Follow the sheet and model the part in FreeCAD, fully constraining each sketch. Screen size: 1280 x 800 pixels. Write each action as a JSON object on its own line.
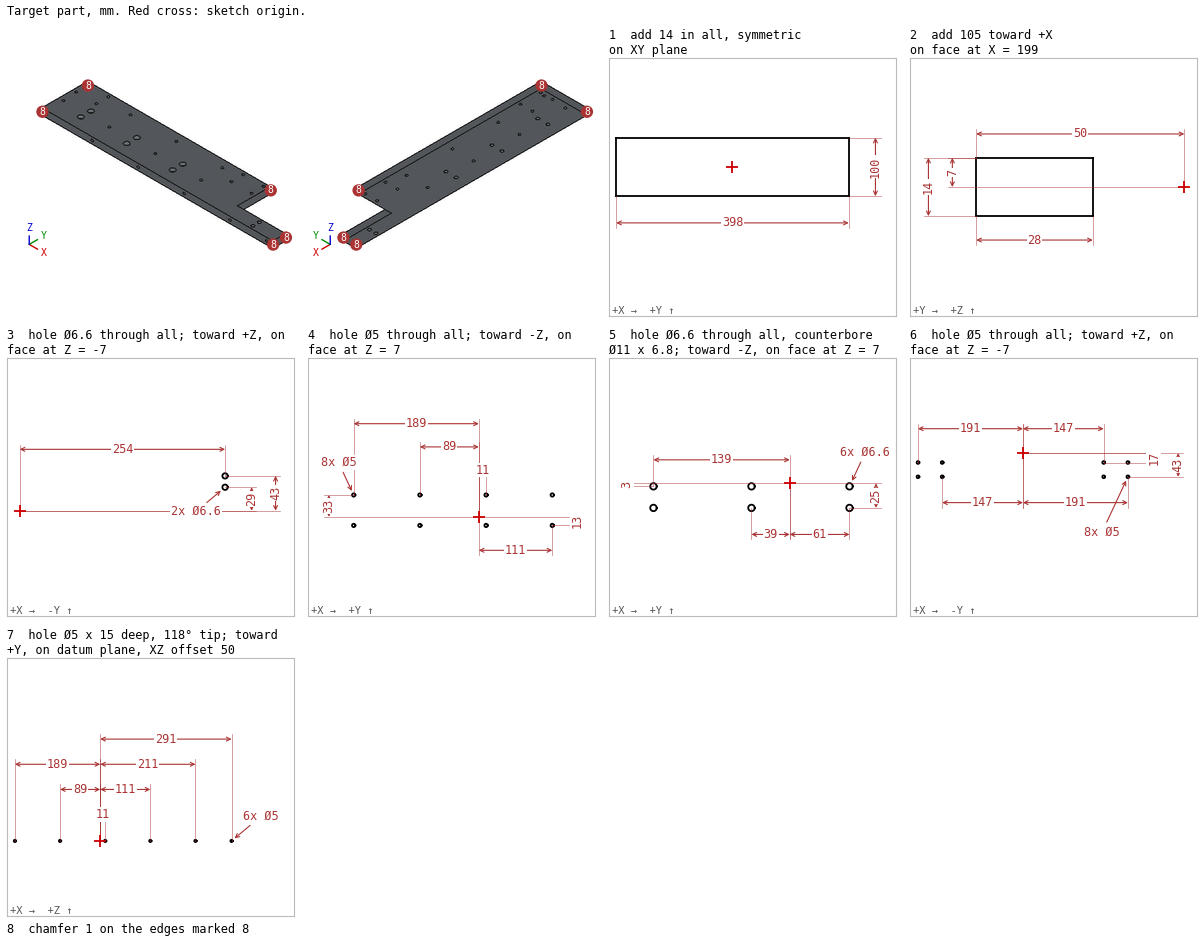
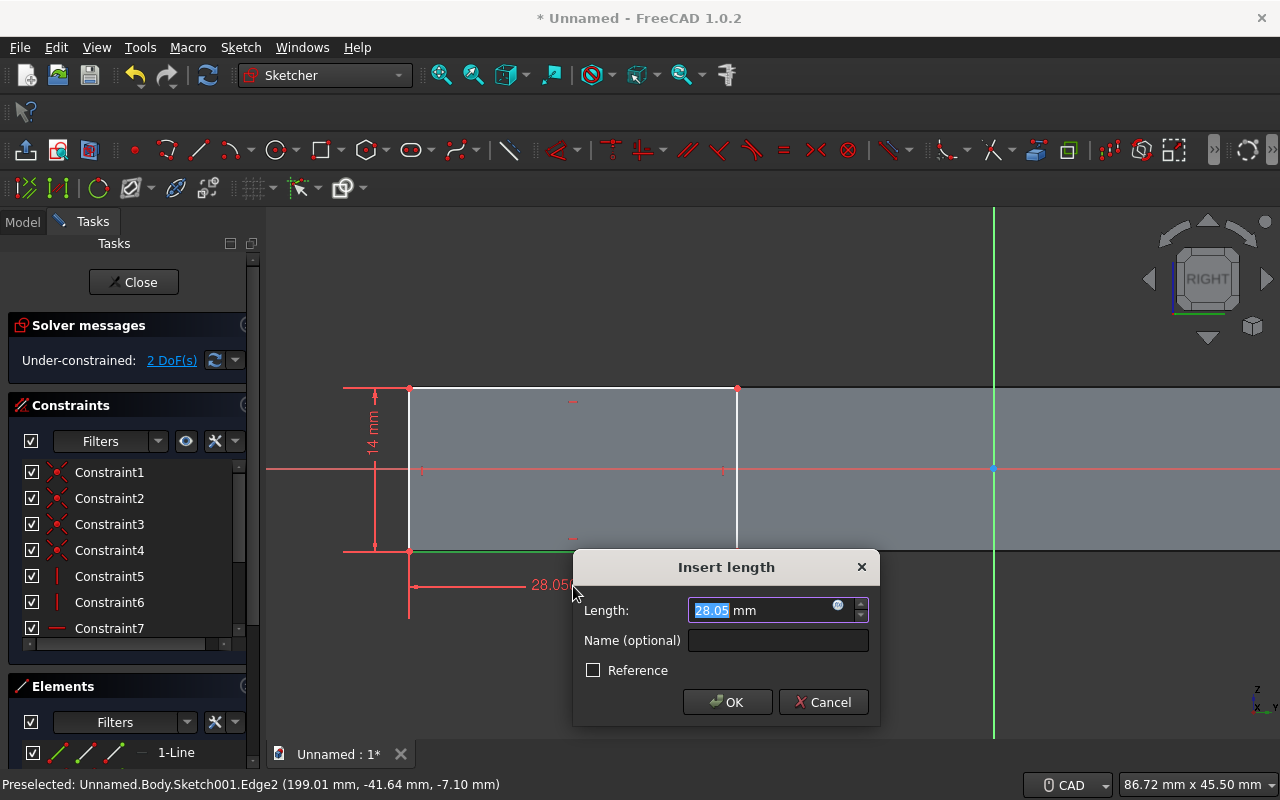
{"action": "type", "text": "28"}
{"action": "key", "text": "Return"}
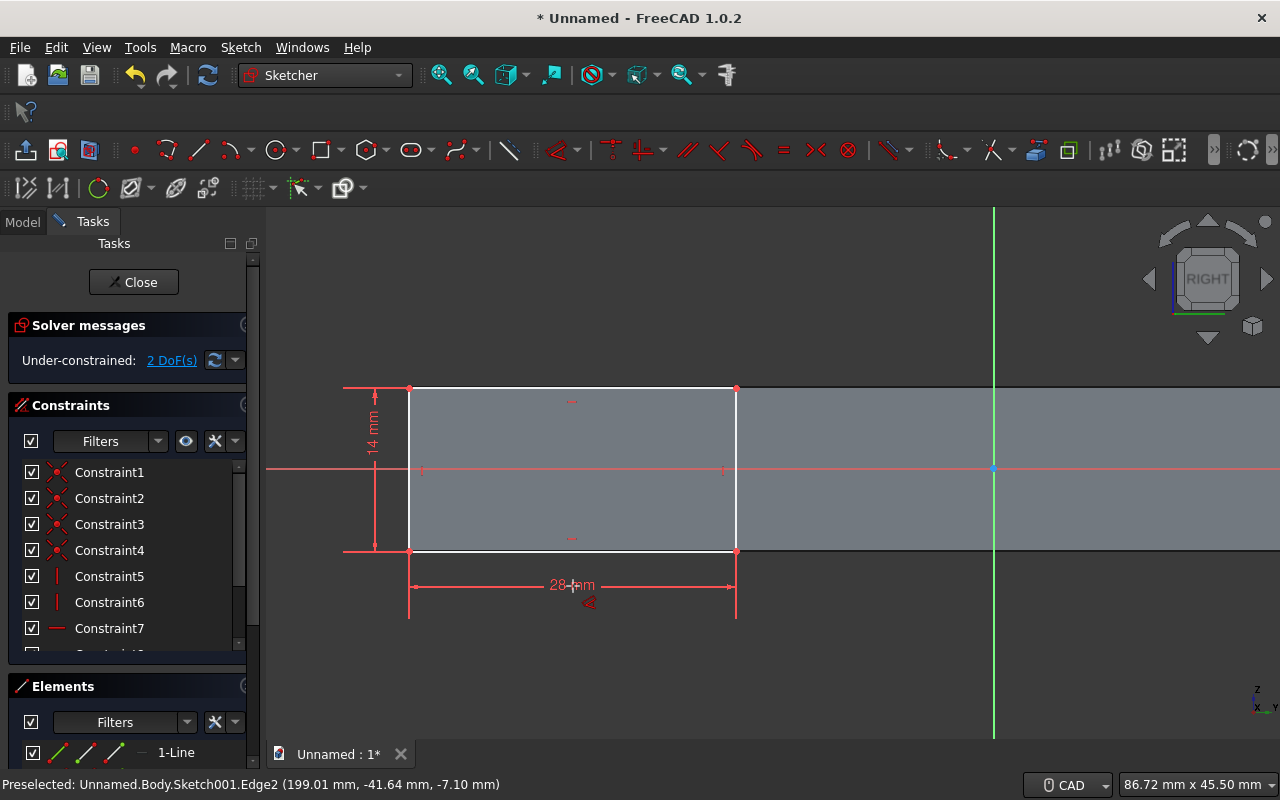
{"action": "left_click", "coordinate": [409, 388]}
{"action": "left_click", "coordinate": [375, 410]}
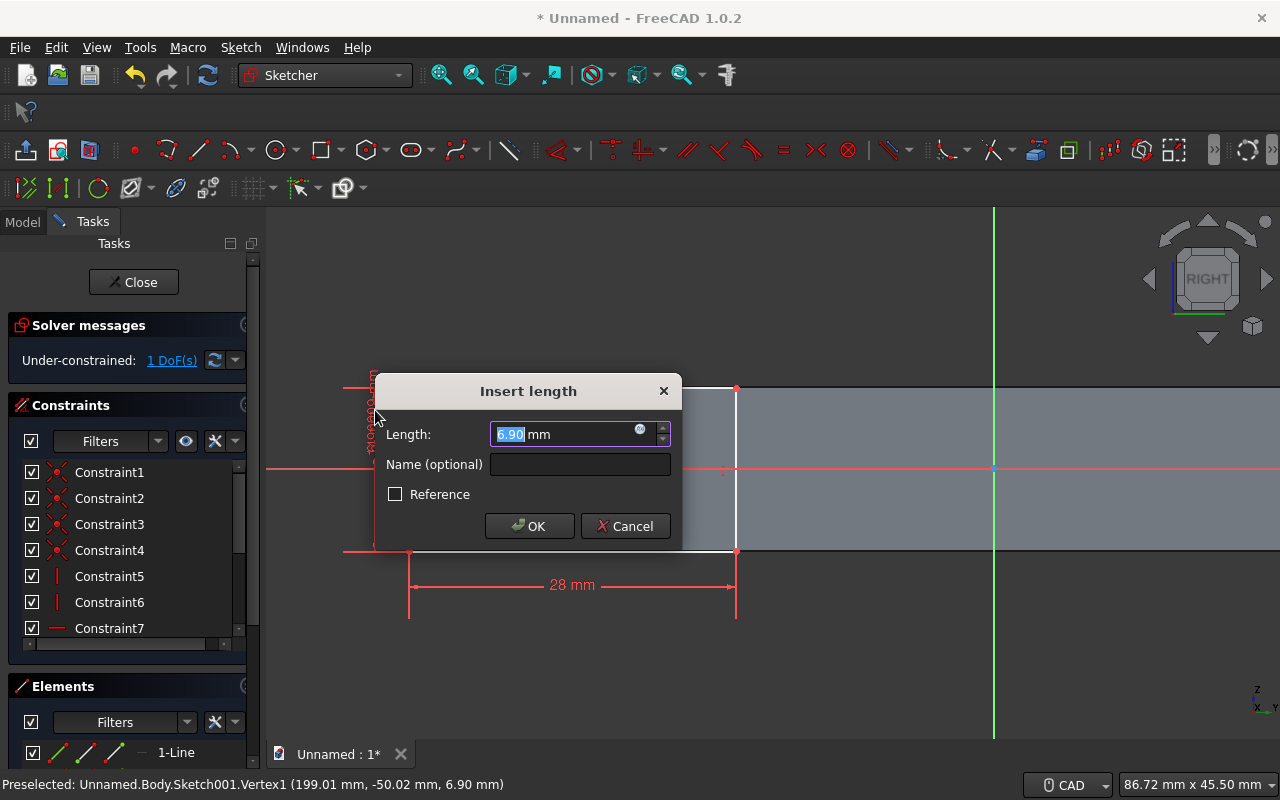
{"action": "type", "text": "7"}
{"action": "key", "text": "Return"}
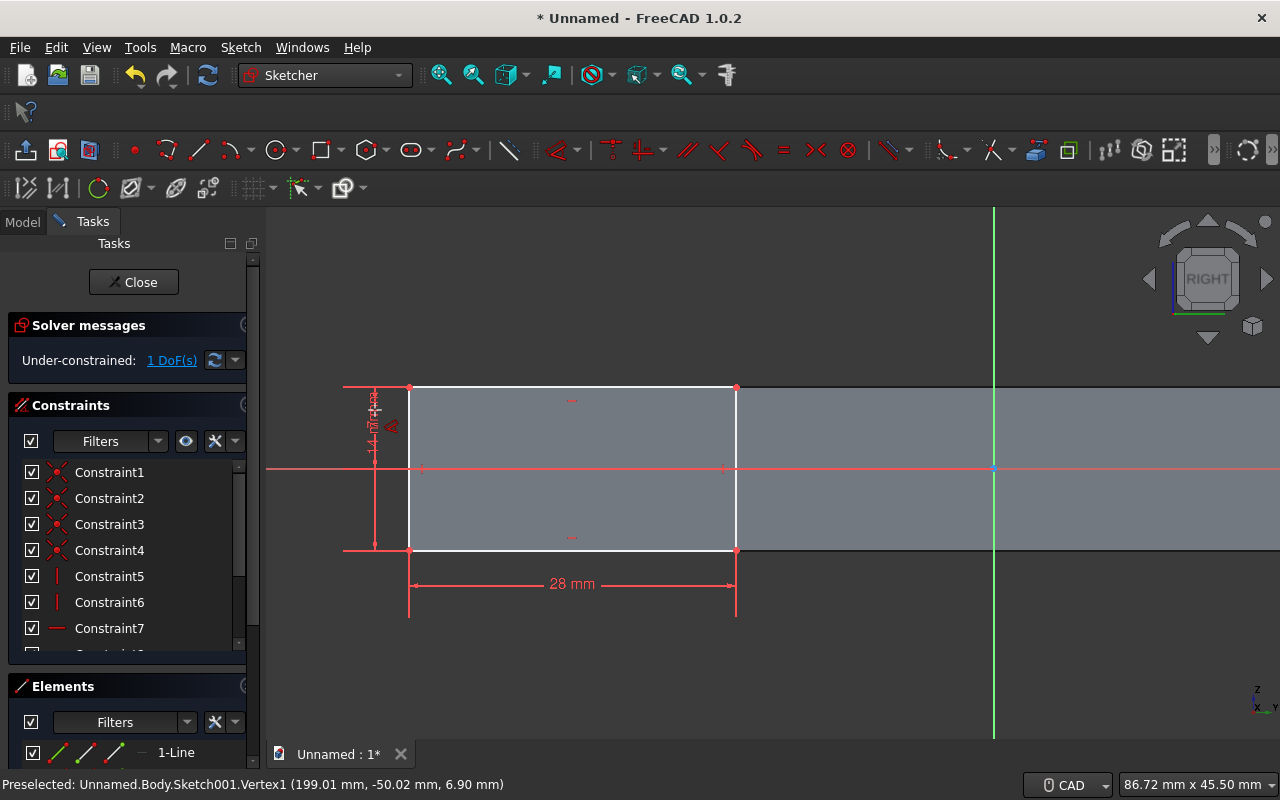
{"action": "left_click", "coordinate": [409, 387]}
{"action": "left_click", "coordinate": [701, 353]}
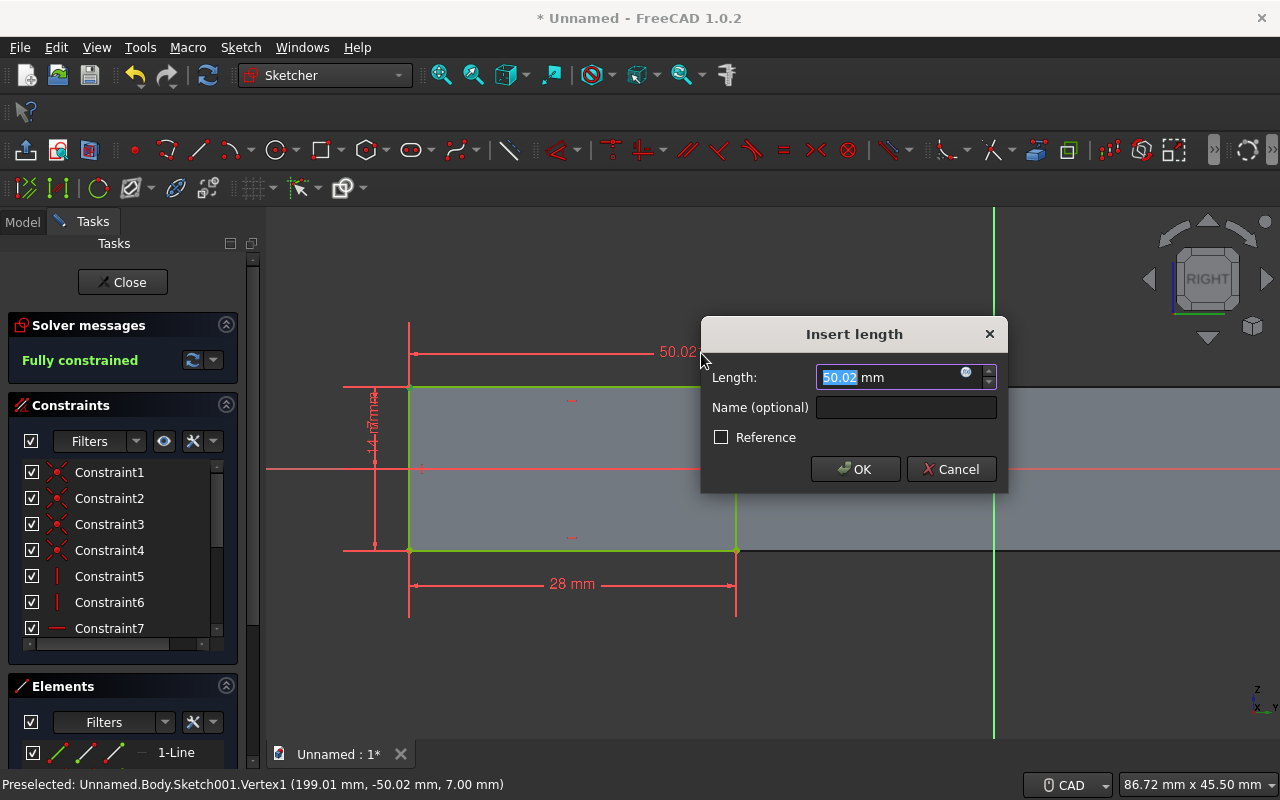
{"action": "type", "text": "50"}
{"action": "key", "text": "Return"}
{"action": "key", "text": "Escape"}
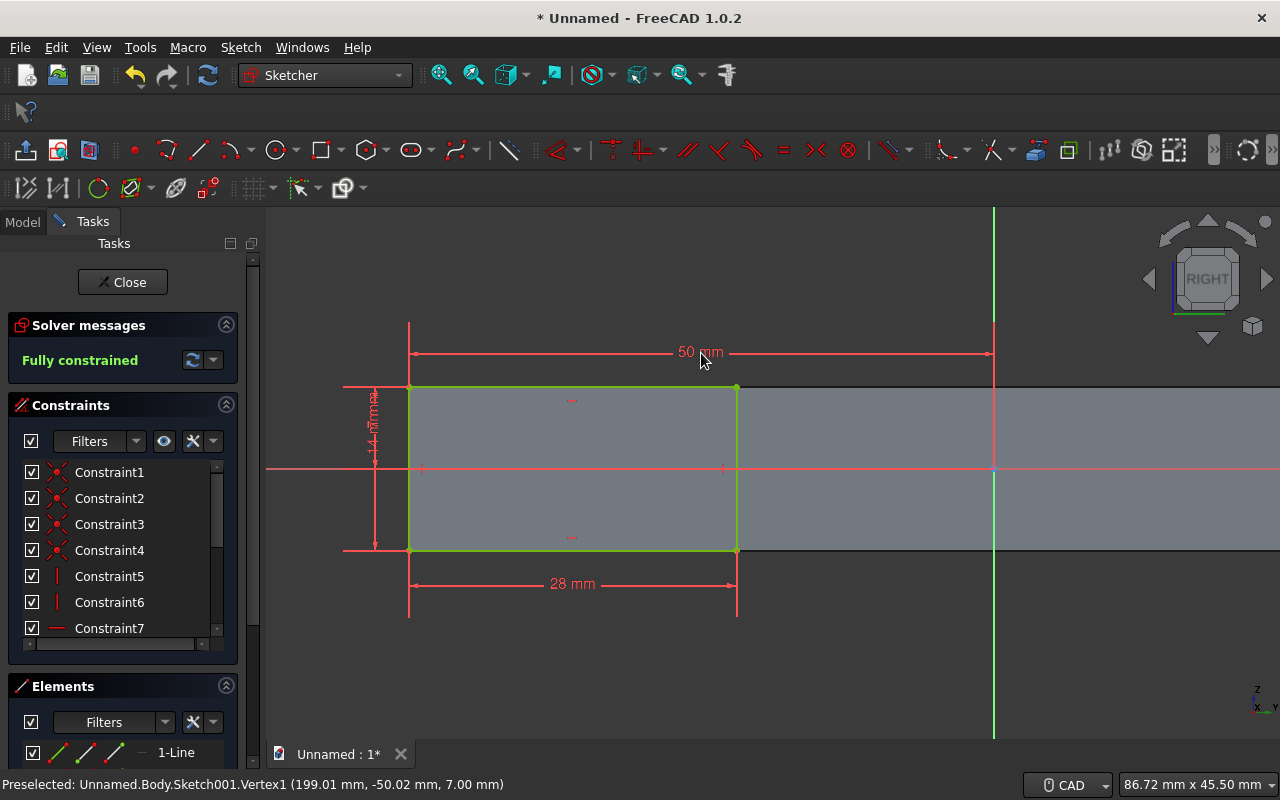
{"action": "left_click", "coordinate": [123, 282]}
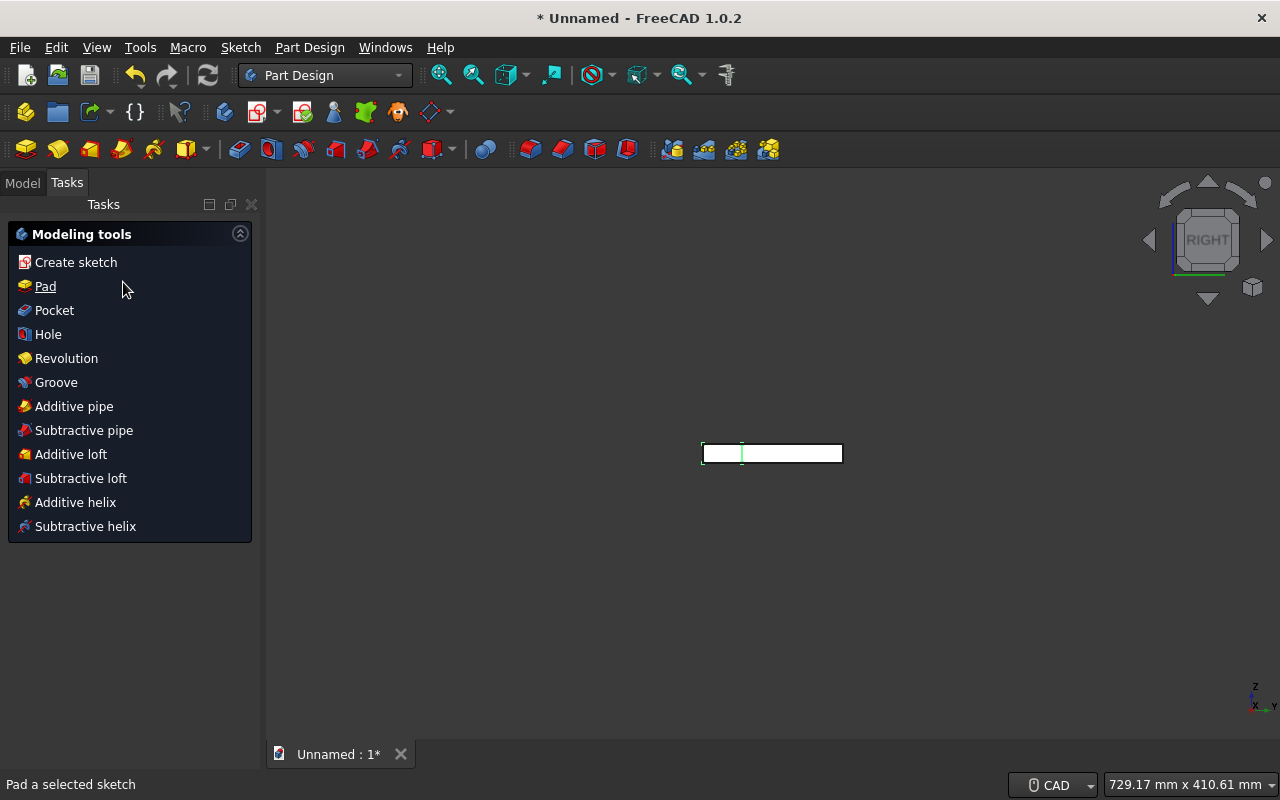
{"action": "left_click", "coordinate": [26, 150]}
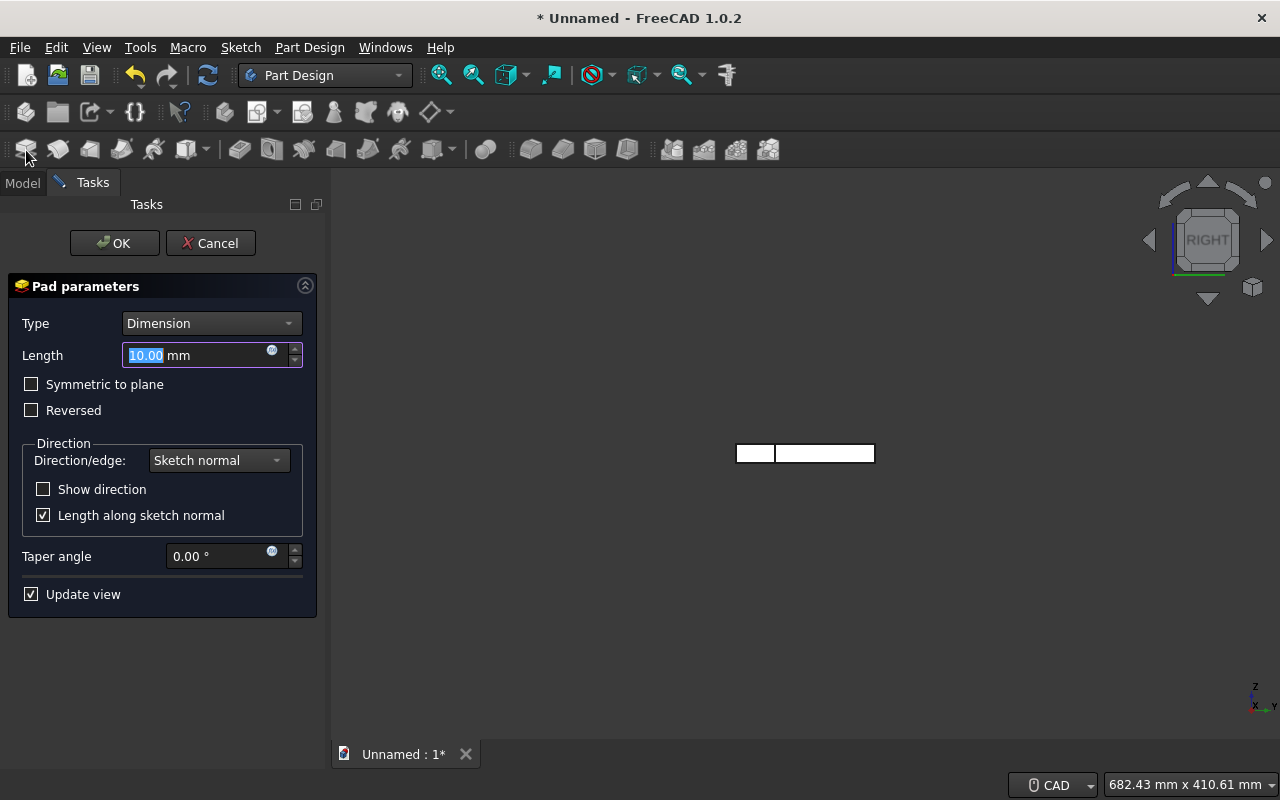
{"action": "type", "text": "105"}
{"action": "key", "text": "Tab"}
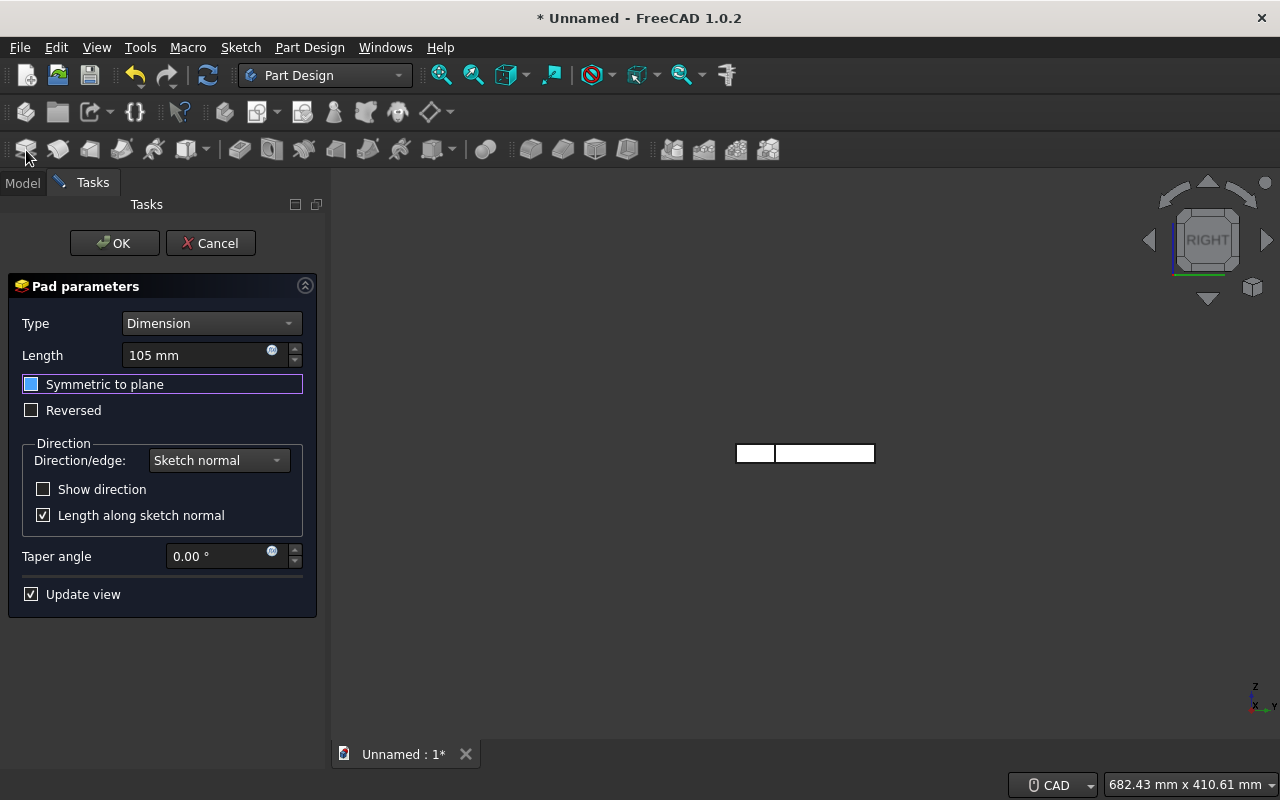
{"action": "left_click", "coordinate": [115, 243]}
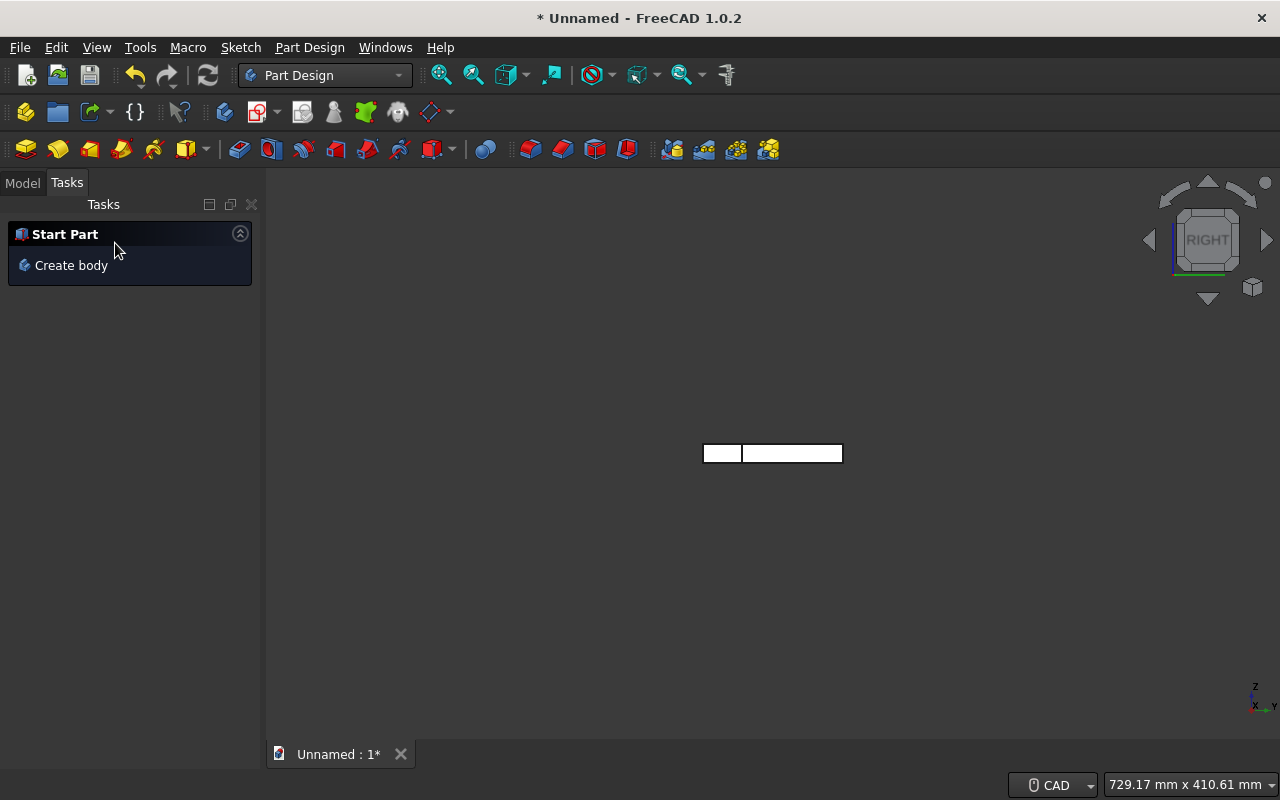
{"action": "key", "text": "v f"}